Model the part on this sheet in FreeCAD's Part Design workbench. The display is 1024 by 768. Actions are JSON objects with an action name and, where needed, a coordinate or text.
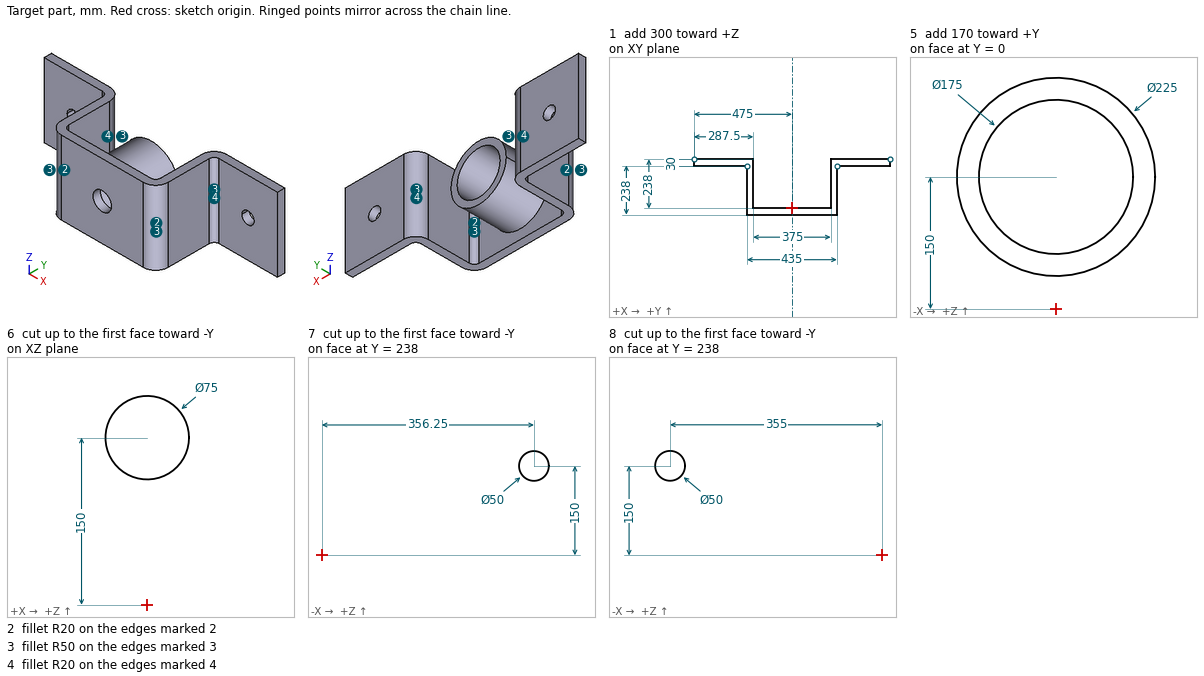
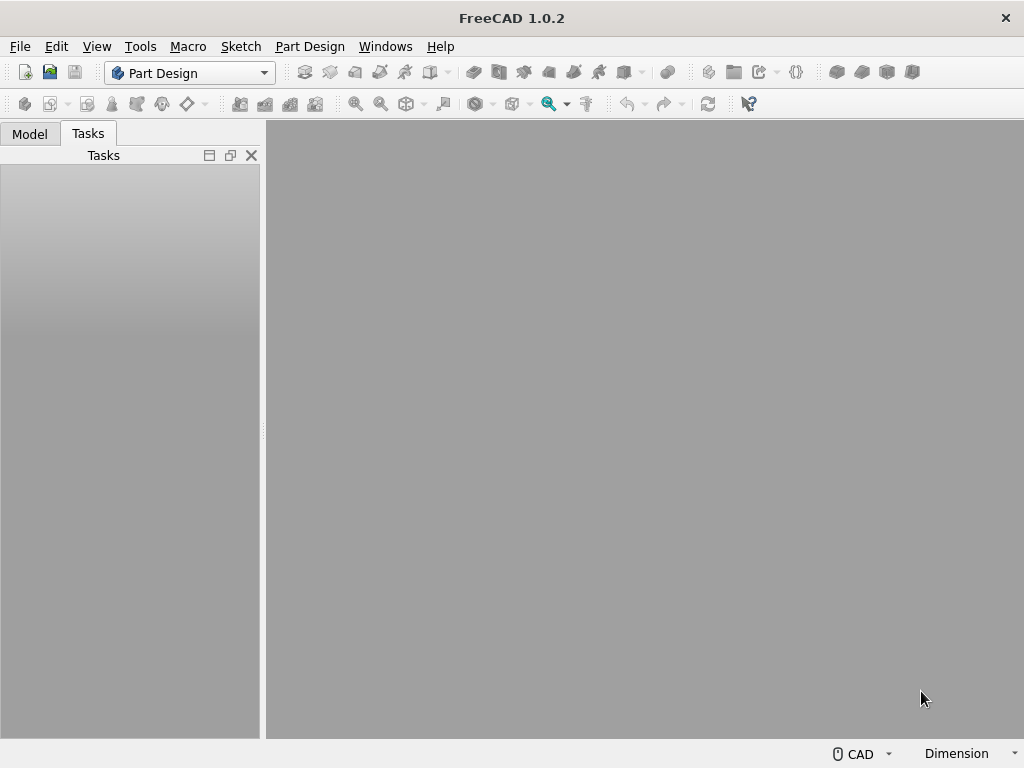
{"action": "left_click", "coordinate": [25, 72]}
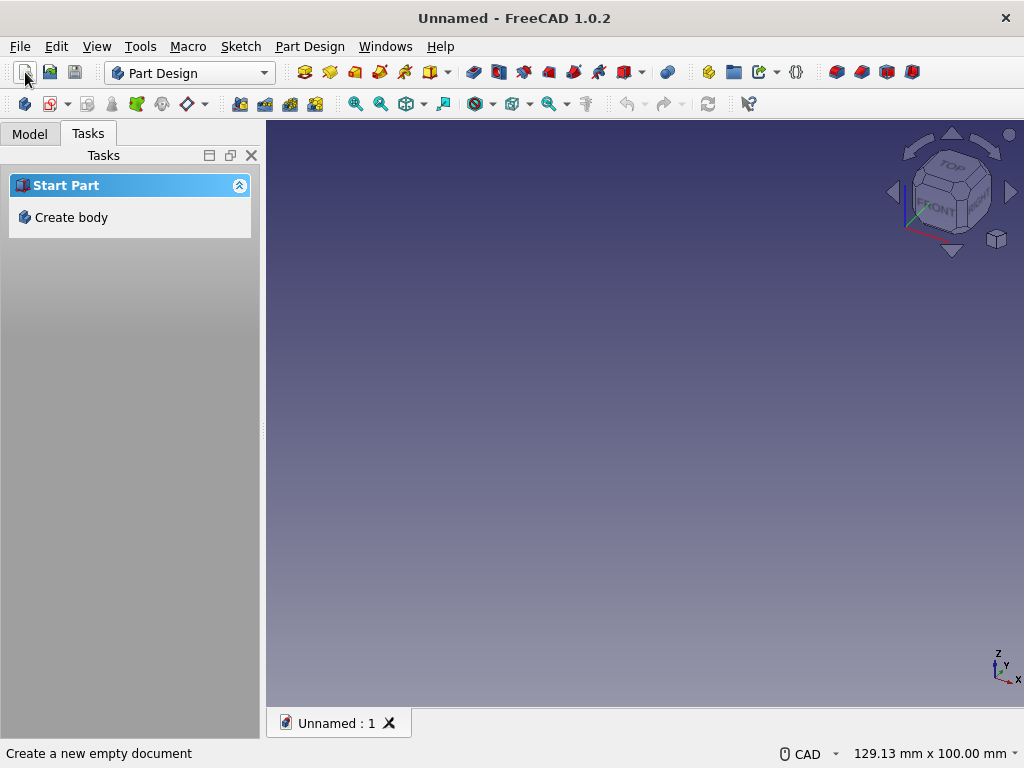
{"action": "left_click", "coordinate": [50, 104]}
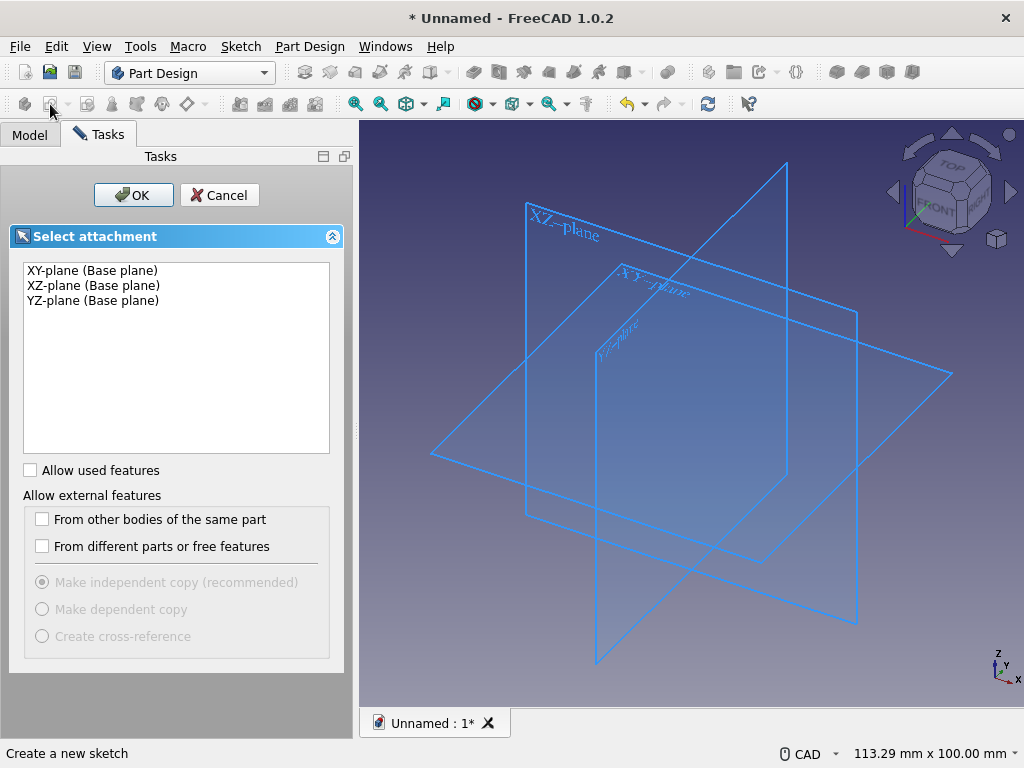
{"action": "left_click", "coordinate": [84, 270]}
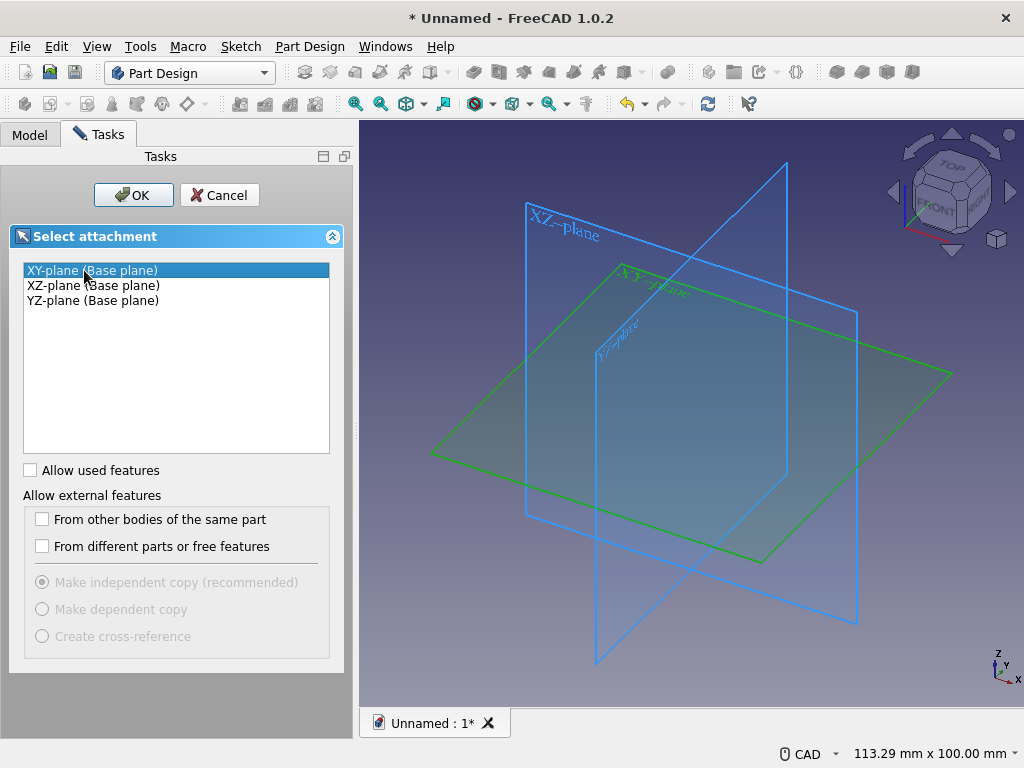
{"action": "left_click", "coordinate": [134, 195]}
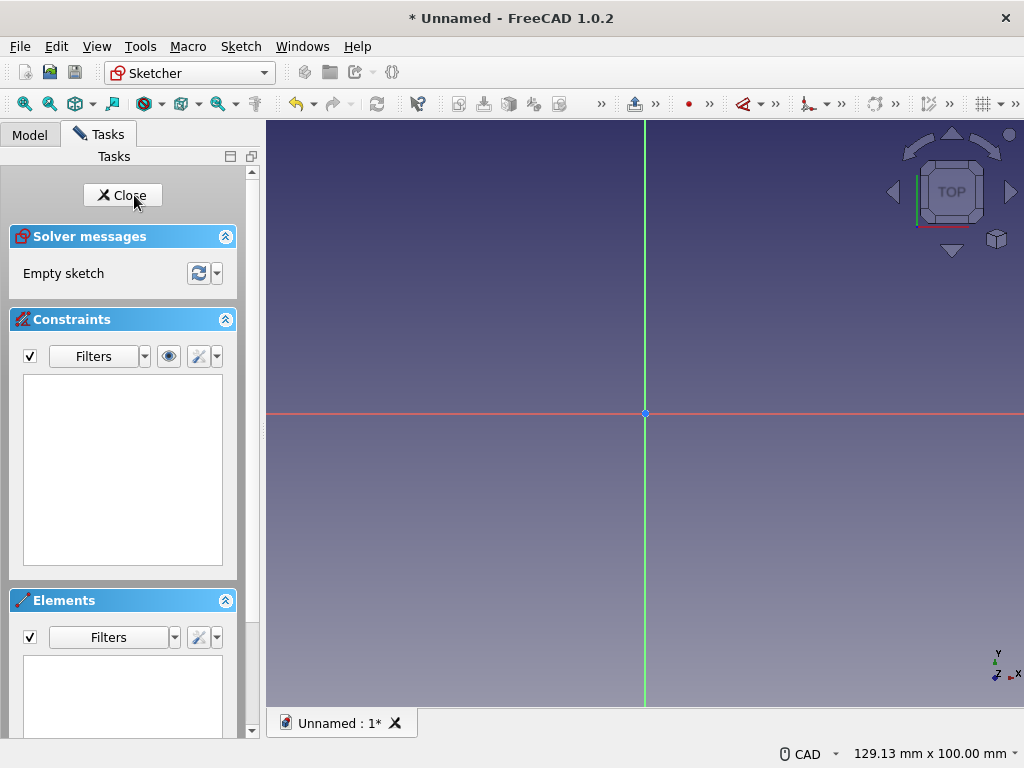
{"action": "scroll", "coordinate": [571, 462], "scroll_direction": "down", "scroll_amount": 13}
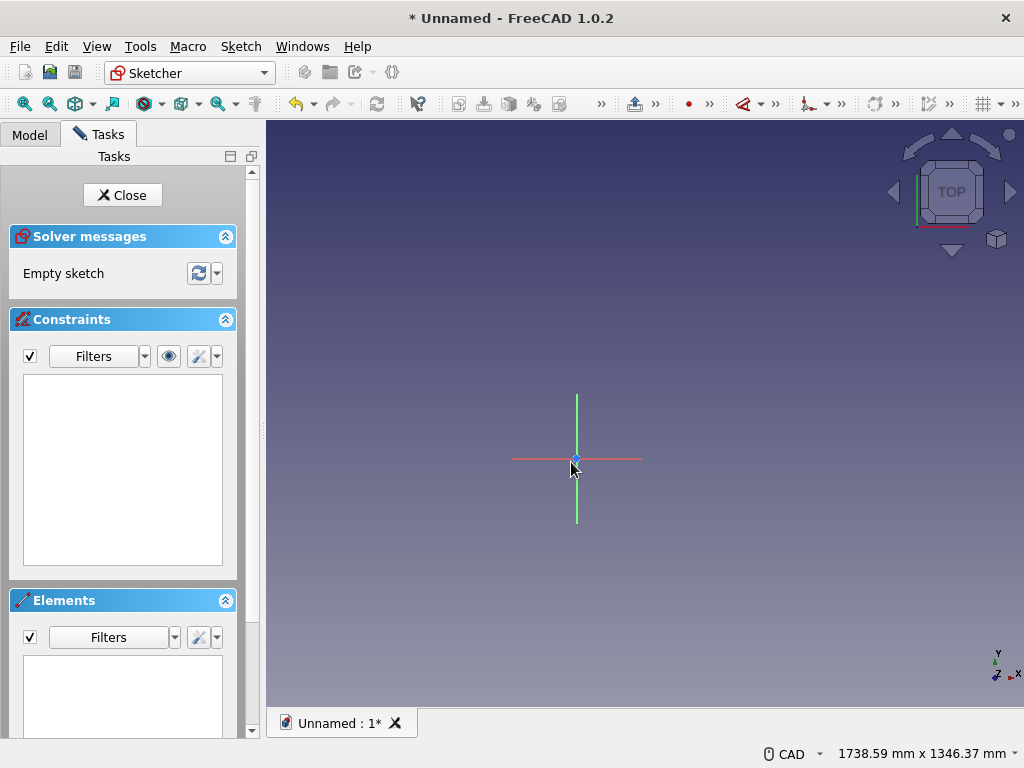
{"action": "key", "text": "g m"}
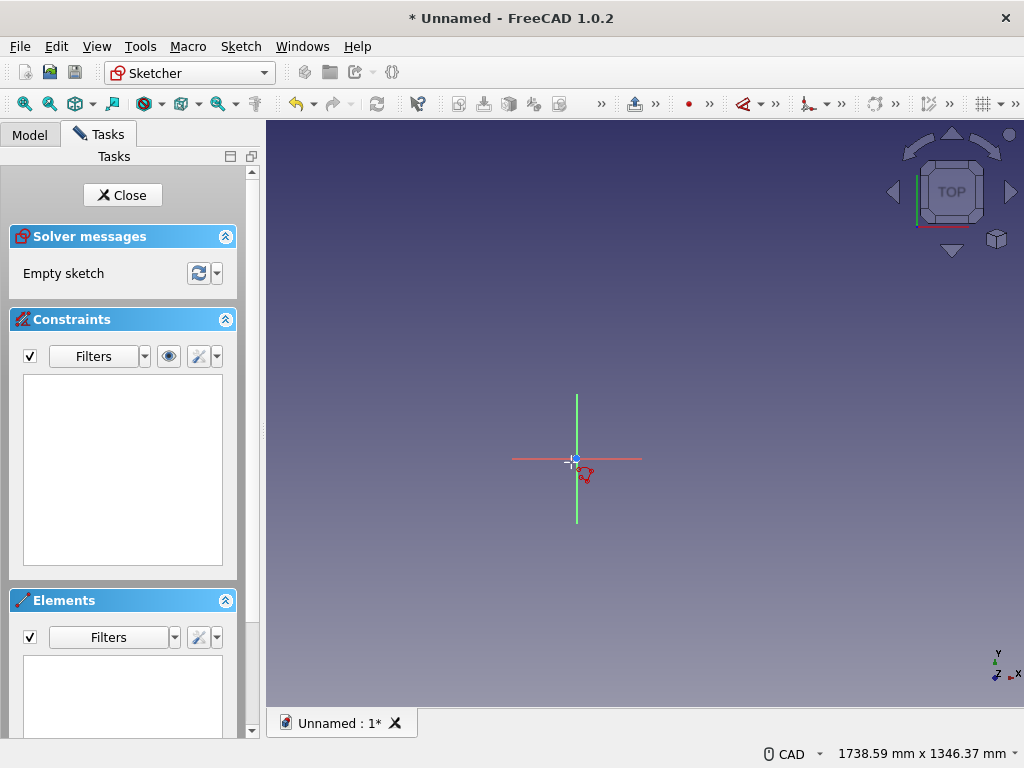
{"action": "left_click", "coordinate": [659, 459]}
{"action": "left_click", "coordinate": [495, 450]}
{"action": "left_click", "coordinate": [495, 355]}
{"action": "left_click", "coordinate": [370, 355]}
{"action": "left_click", "coordinate": [370, 368]}
{"action": "left_click", "coordinate": [482, 368]}
{"action": "left_click", "coordinate": [482, 472]}
{"action": "left_click", "coordinate": [672, 472]}
{"action": "left_click", "coordinate": [672, 368]}
{"action": "left_click", "coordinate": [784, 368]}
{"action": "left_click", "coordinate": [784, 355]}
{"action": "left_click", "coordinate": [659, 355]}
{"action": "left_click", "coordinate": [659, 460]}
{"action": "key", "text": "Escape"}
{"action": "key", "text": "Escape"}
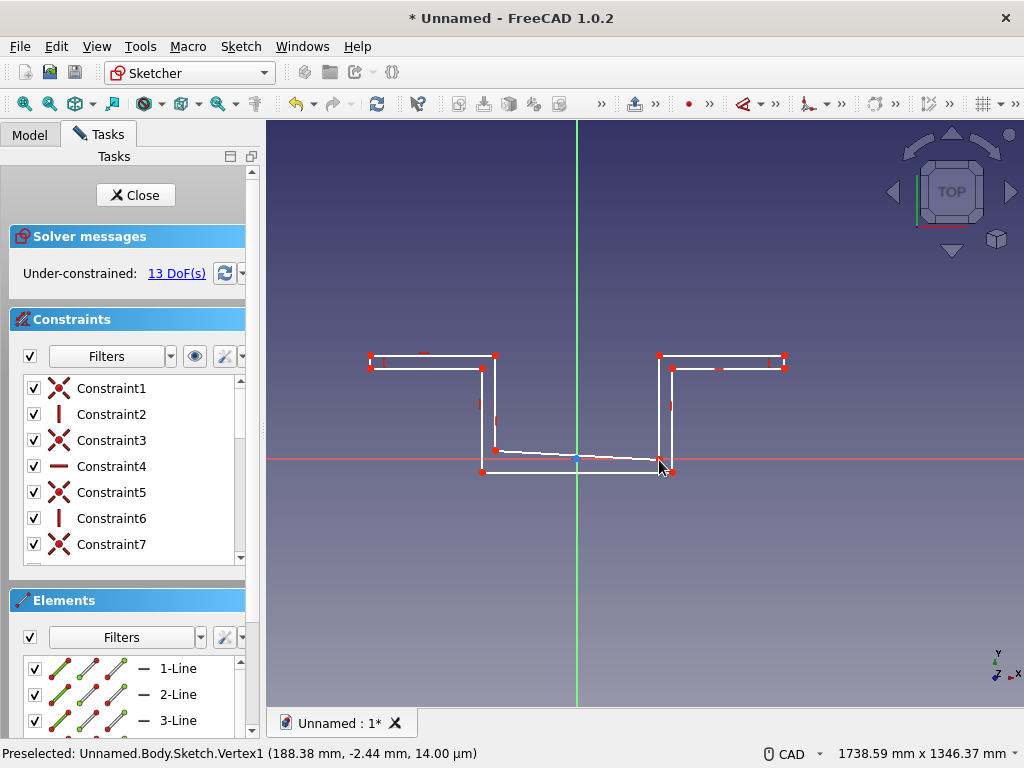
{"action": "left_click", "coordinate": [610, 457]}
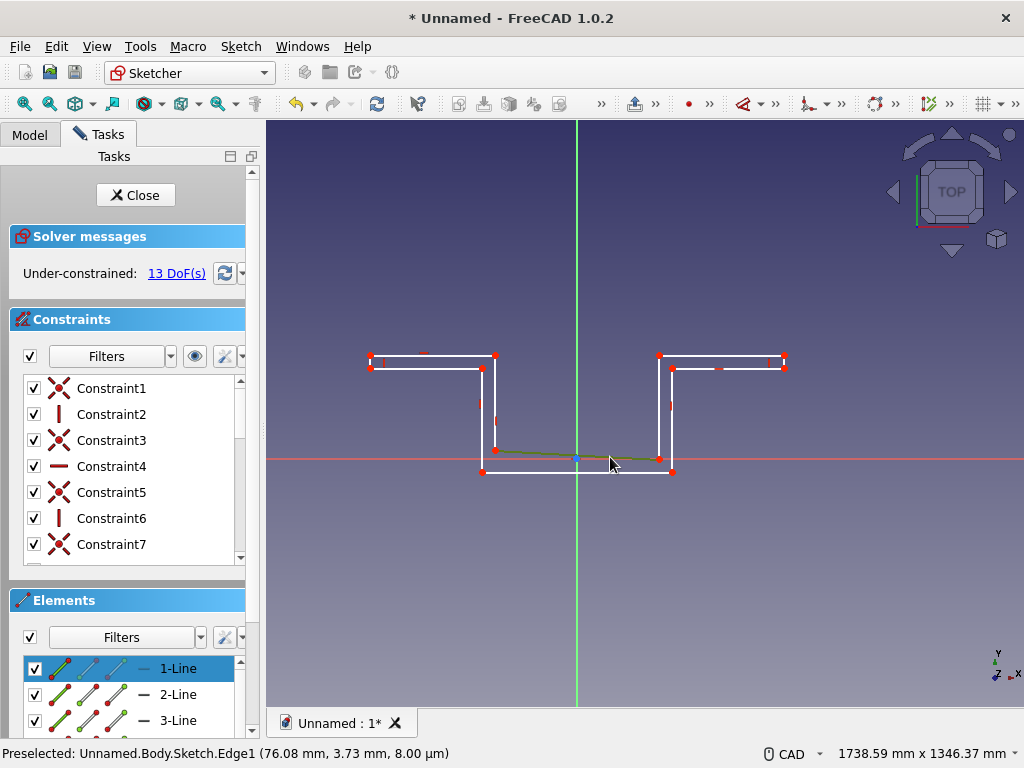
{"action": "key", "text": "h"}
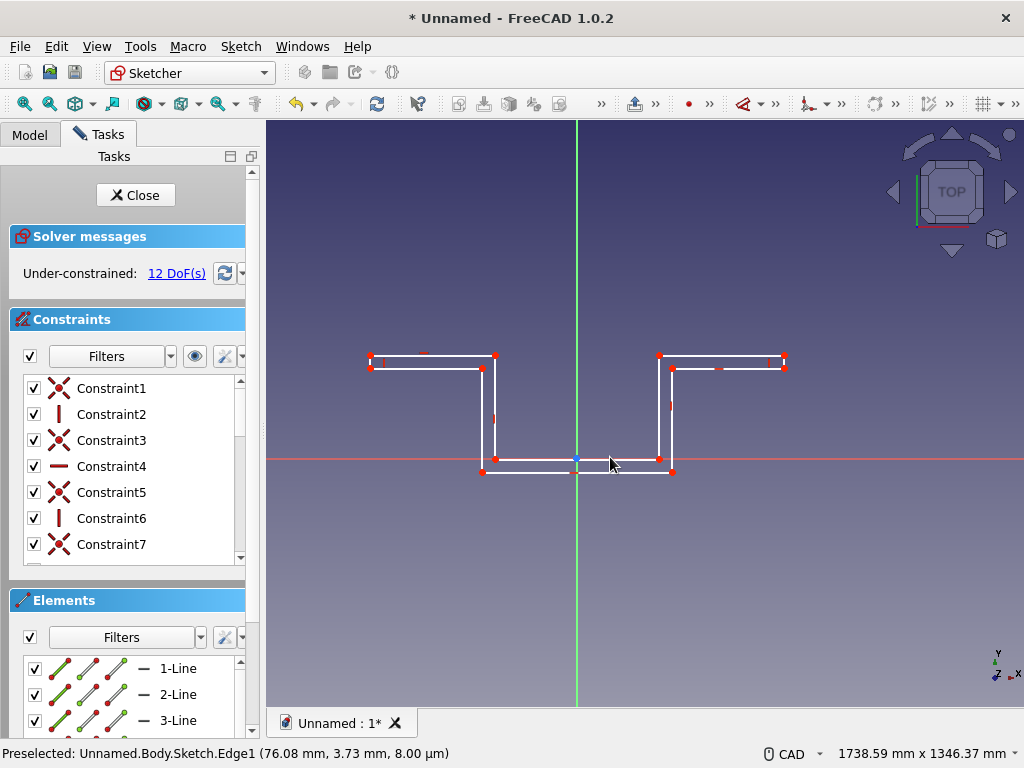
{"action": "left_click", "coordinate": [482, 369]}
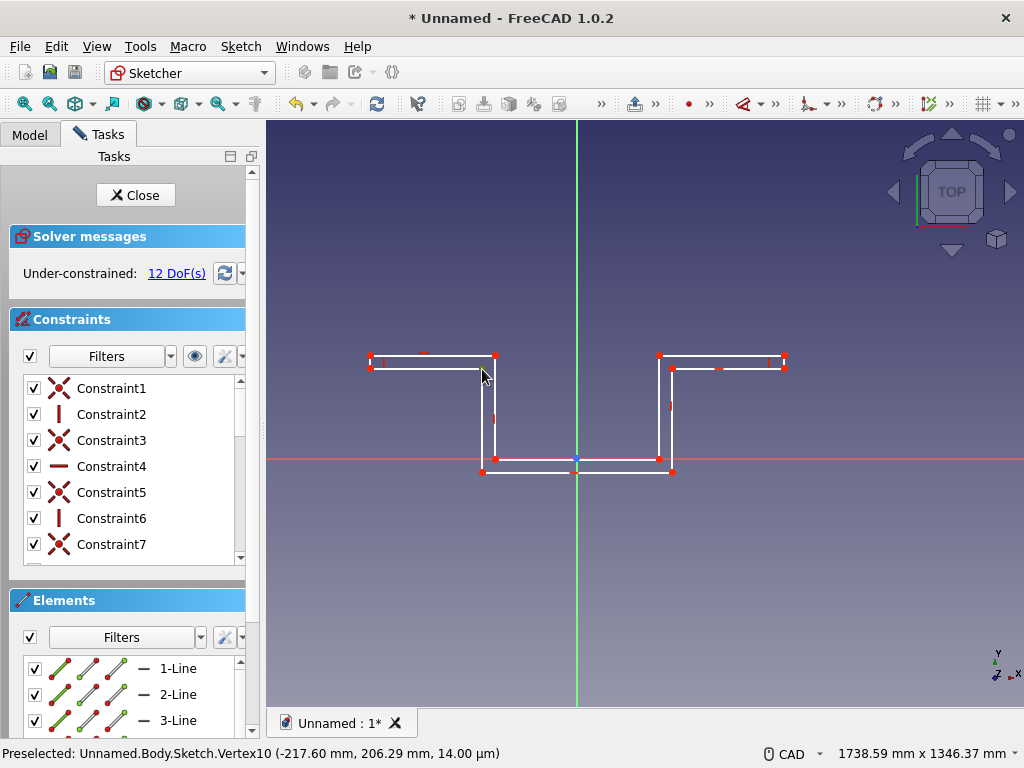
{"action": "left_click", "coordinate": [672, 369]}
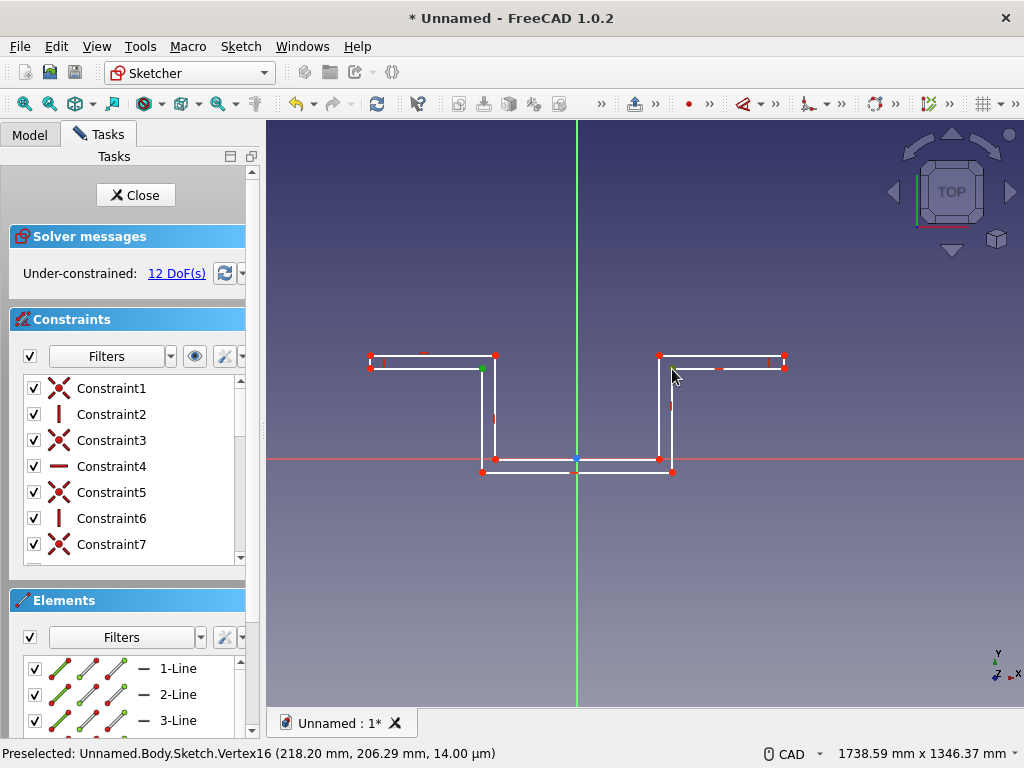
{"action": "left_click", "coordinate": [577, 641]}